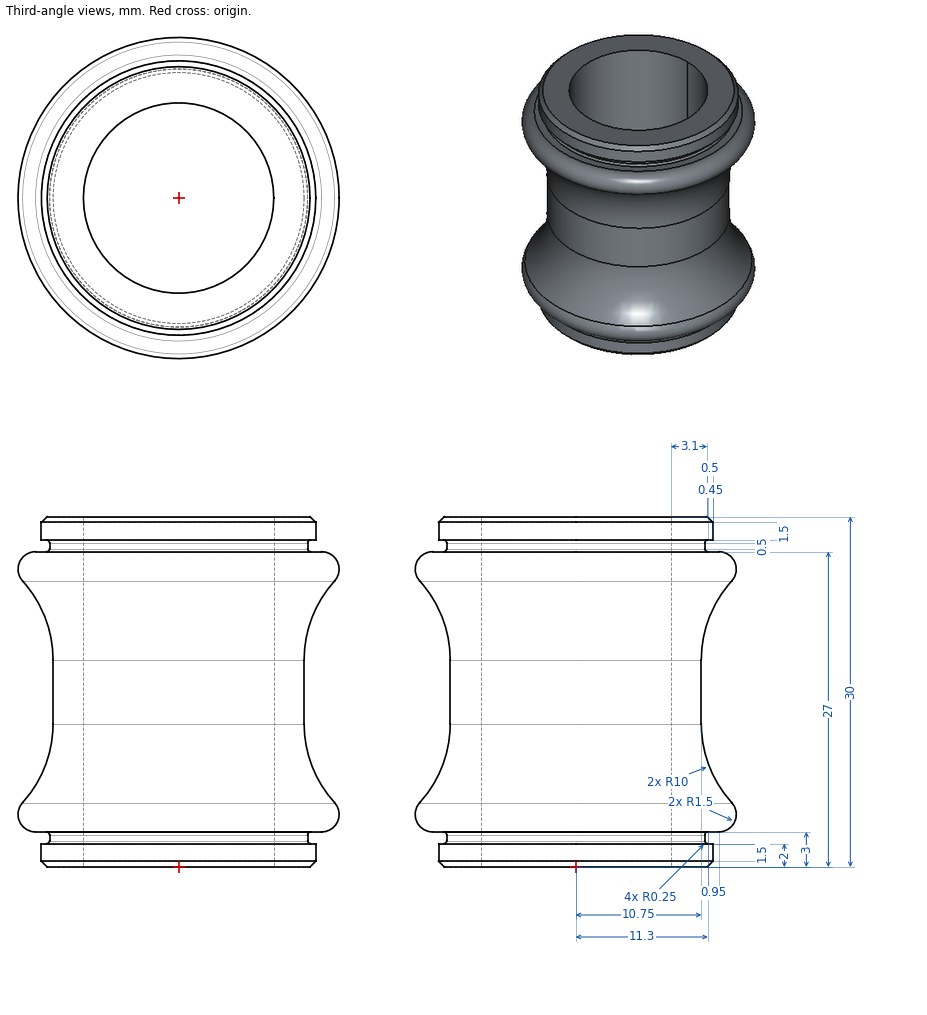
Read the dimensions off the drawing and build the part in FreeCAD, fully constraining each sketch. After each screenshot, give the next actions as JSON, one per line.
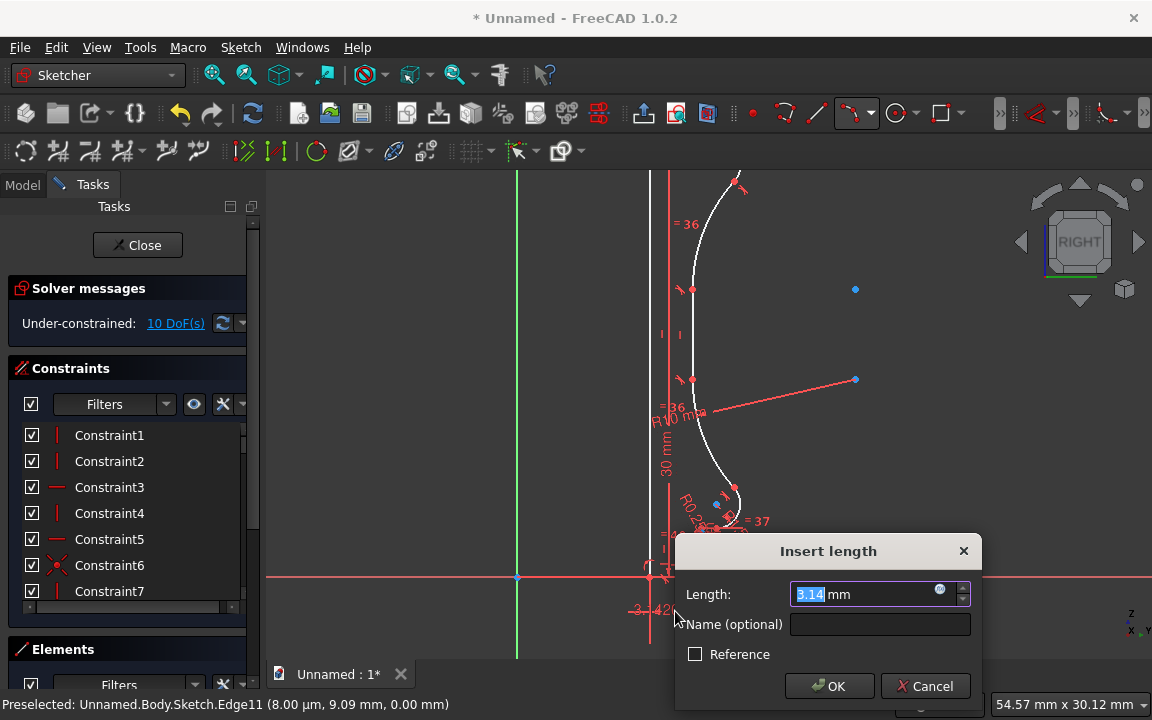
{"action": "type", "text": "3.1"}
{"action": "key", "text": "Return"}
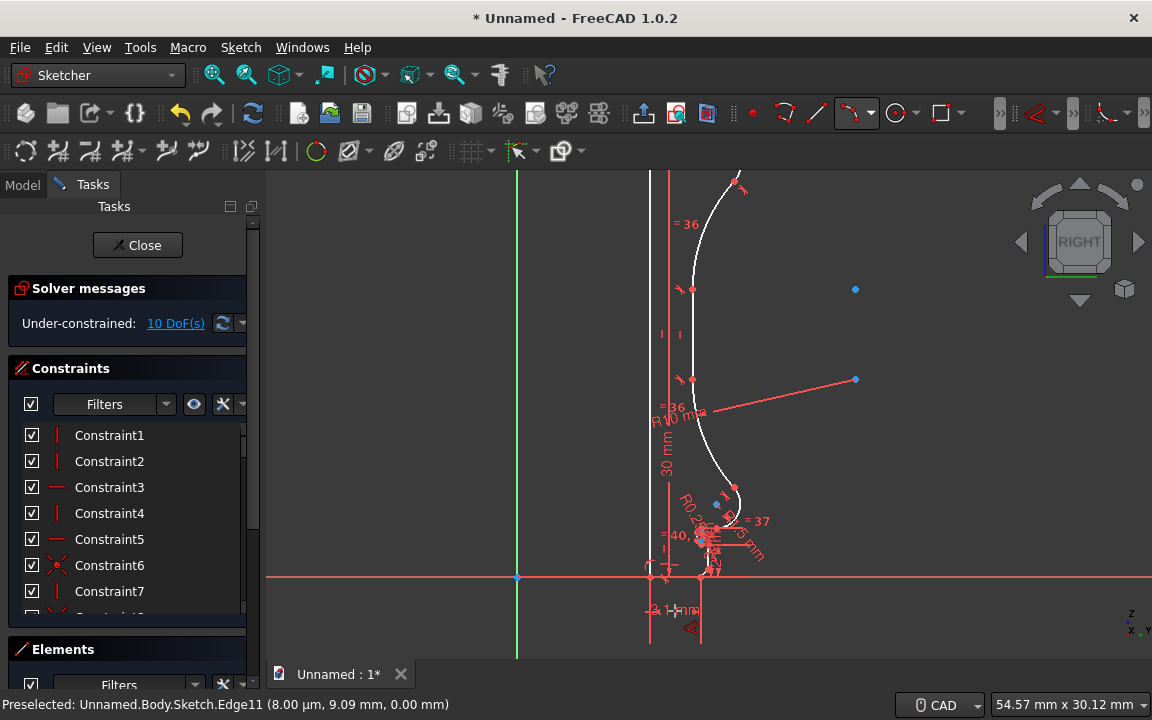
{"action": "scroll", "coordinate": [708, 559], "scroll_direction": "up", "scroll_amount": 3}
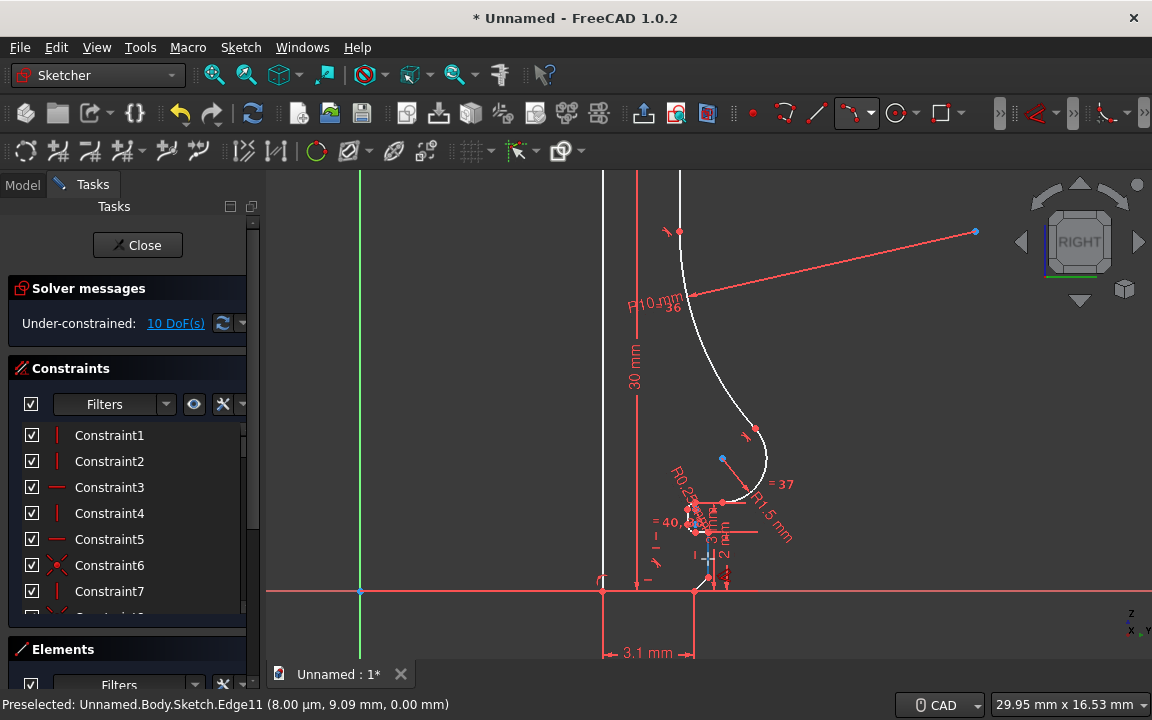
{"action": "left_click", "coordinate": [708, 559]}
{"action": "left_click", "coordinate": [742, 565]}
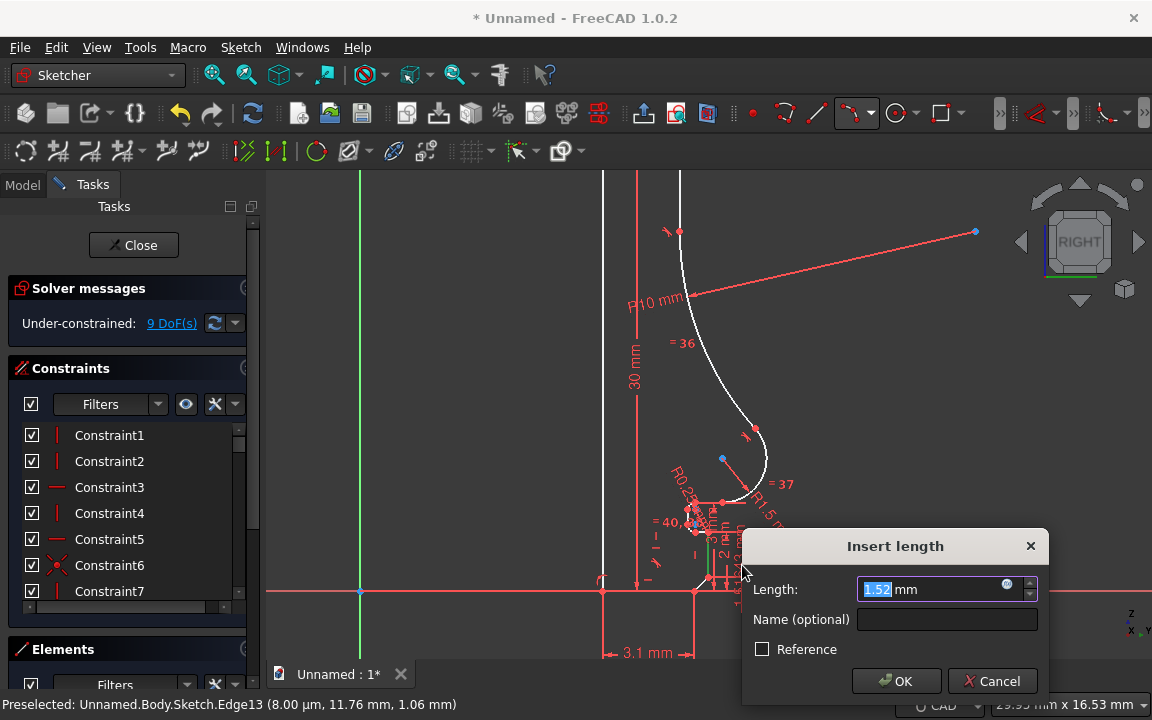
{"action": "type", "text": "1.5"}
{"action": "key", "text": "Return"}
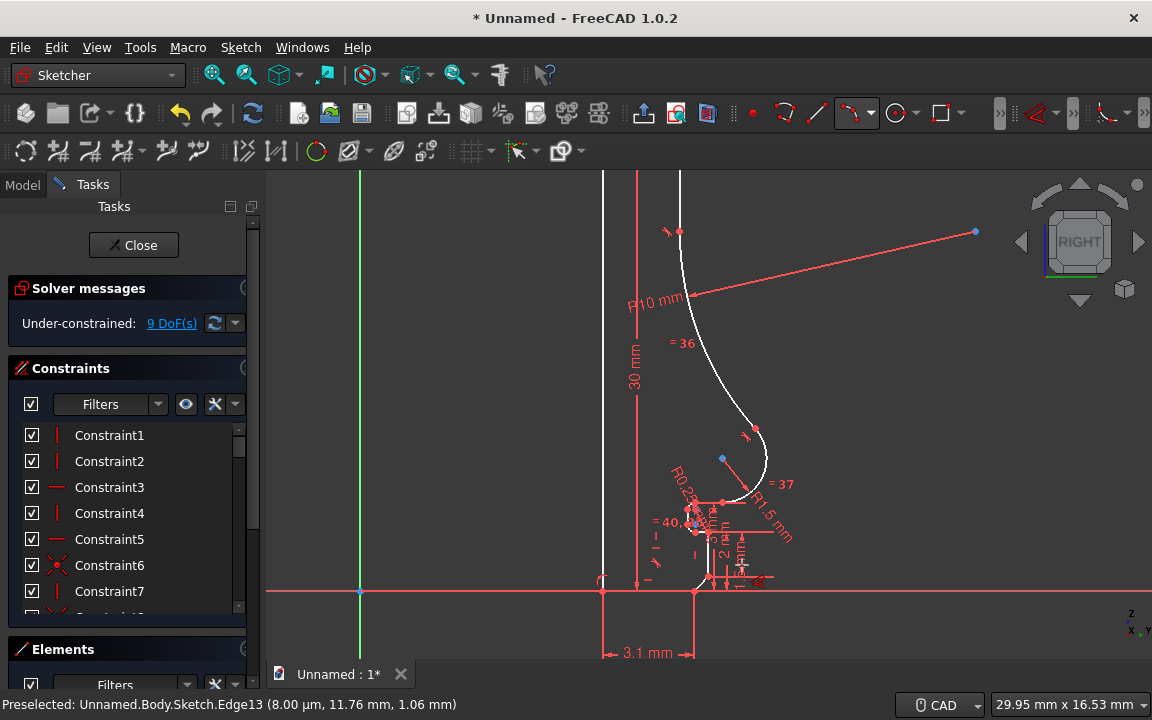
{"action": "scroll", "coordinate": [686, 570], "scroll_direction": "down", "scroll_amount": 5}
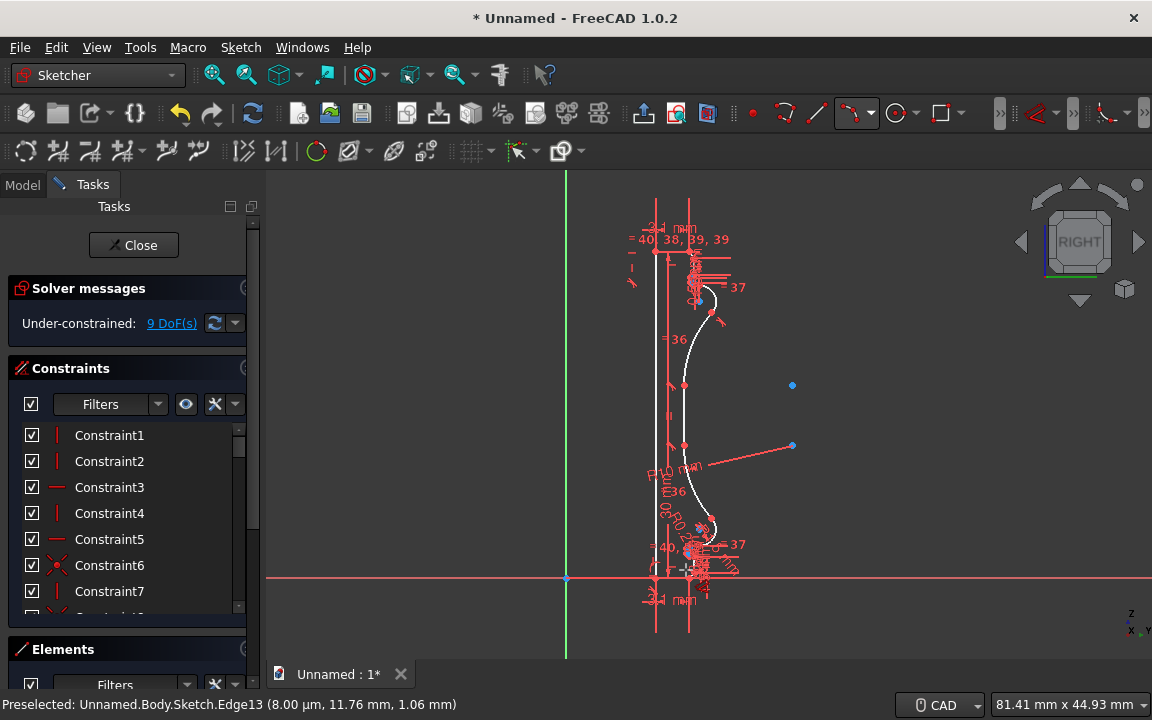
{"action": "scroll", "coordinate": [700, 286], "scroll_direction": "up", "scroll_amount": 4}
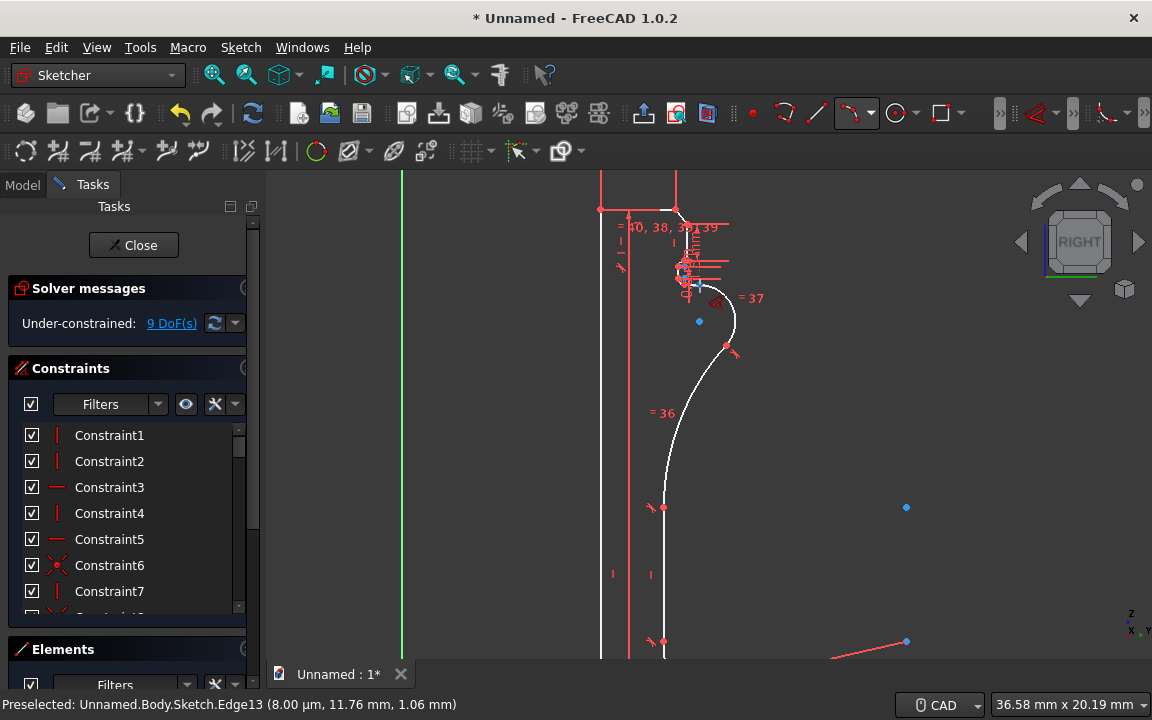
{"action": "left_click", "coordinate": [699, 285]}
{"action": "left_click", "coordinate": [368, 458]}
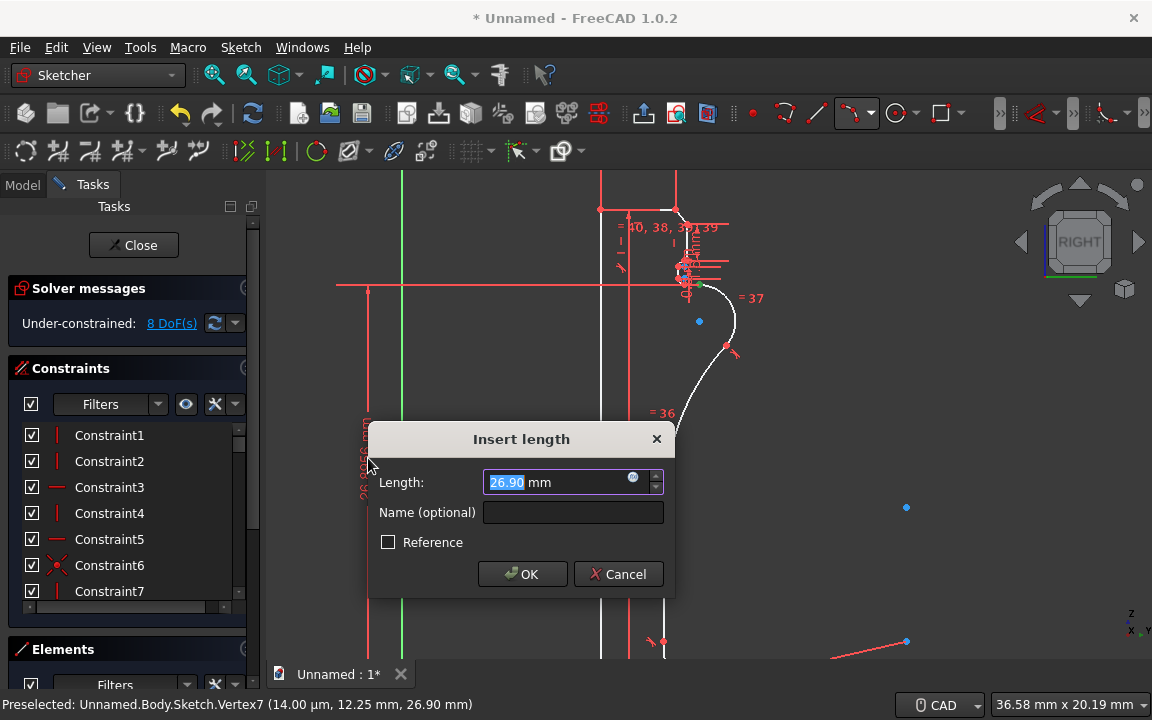
{"action": "type", "text": "27"}
{"action": "key", "text": "Return"}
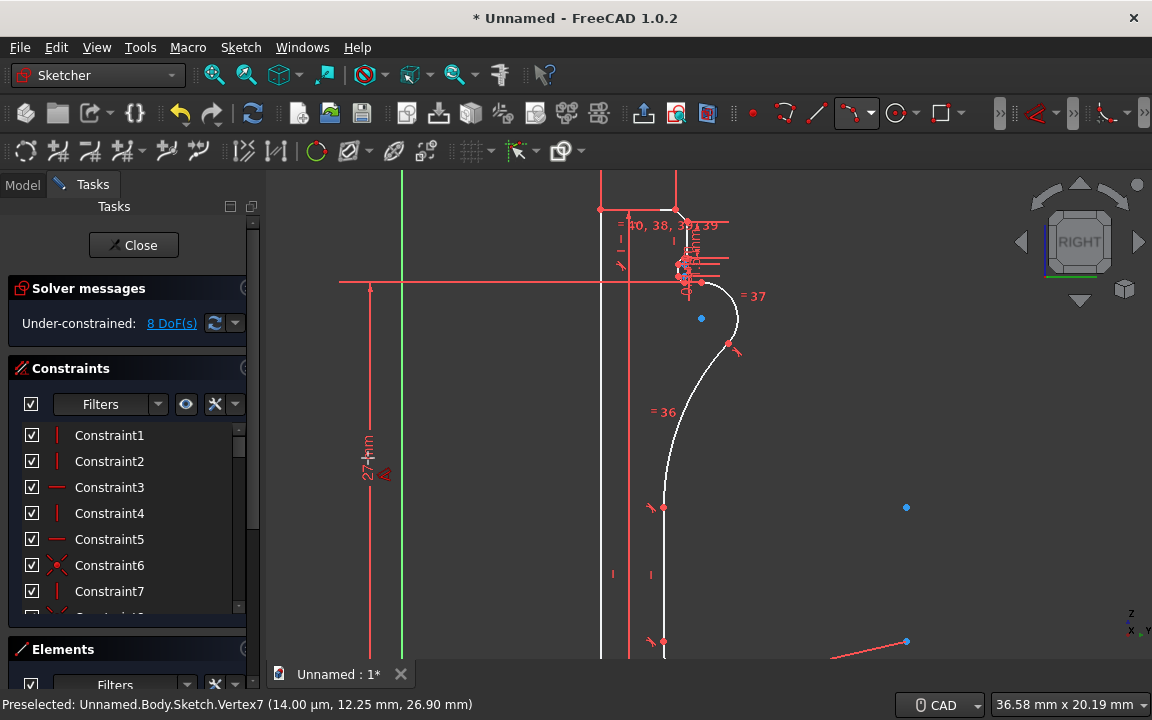
{"action": "scroll", "coordinate": [700, 285], "scroll_direction": "down", "scroll_amount": 4}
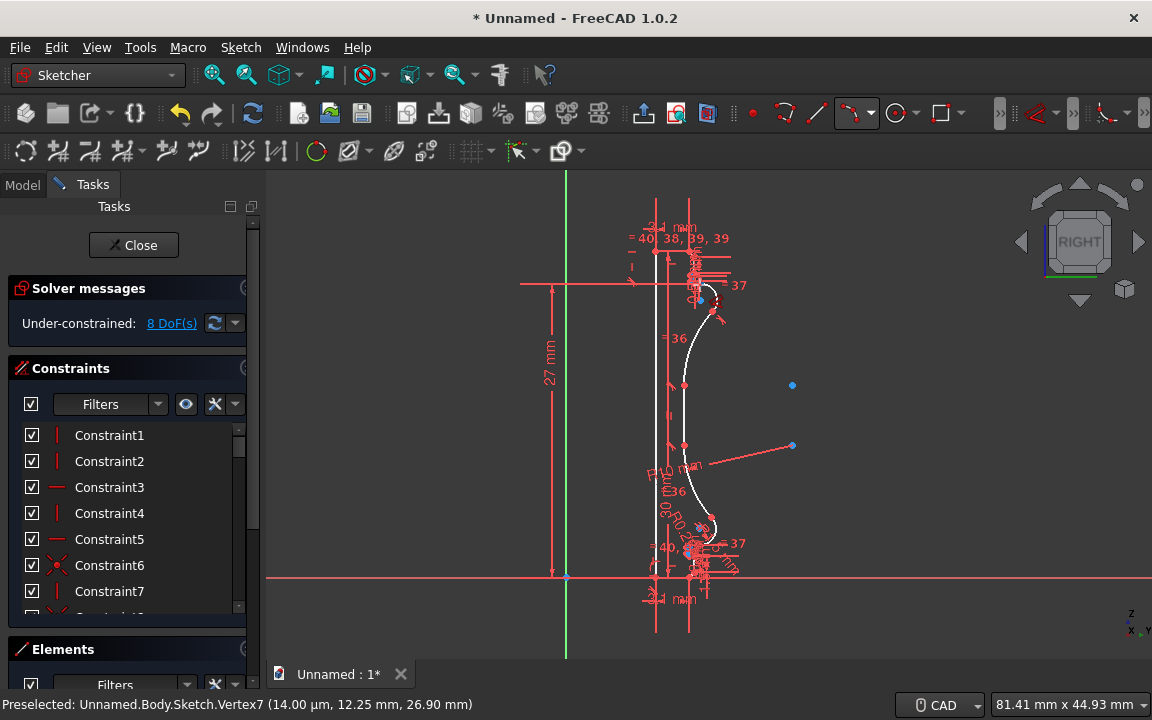
{"action": "scroll", "coordinate": [695, 545], "scroll_direction": "up", "scroll_amount": 7}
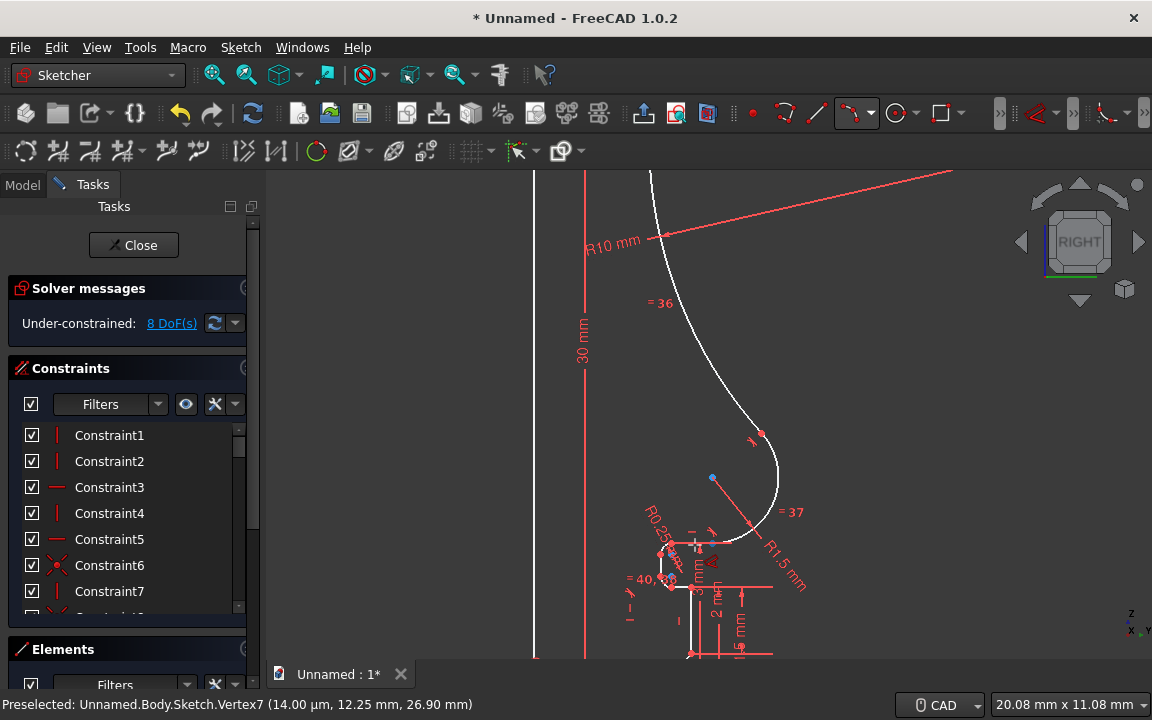
{"action": "left_click", "coordinate": [692, 543]}
{"action": "left_click", "coordinate": [692, 509]}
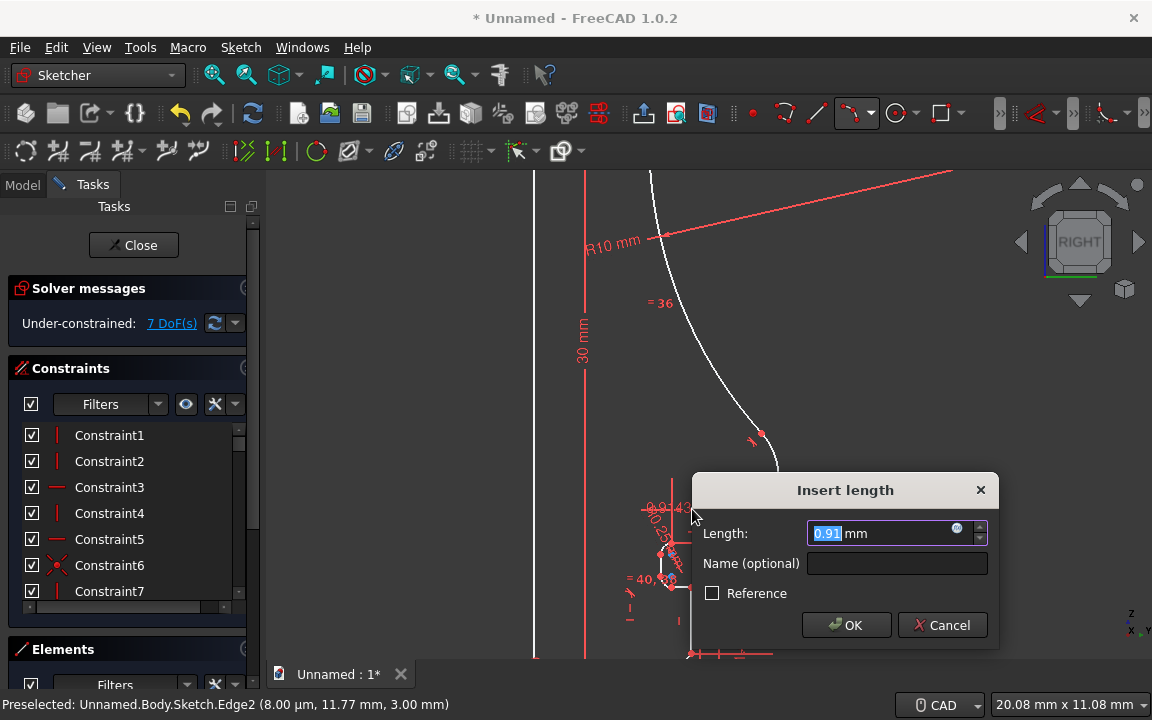
{"action": "type", "text": "0.95"}
{"action": "key", "text": "Return"}